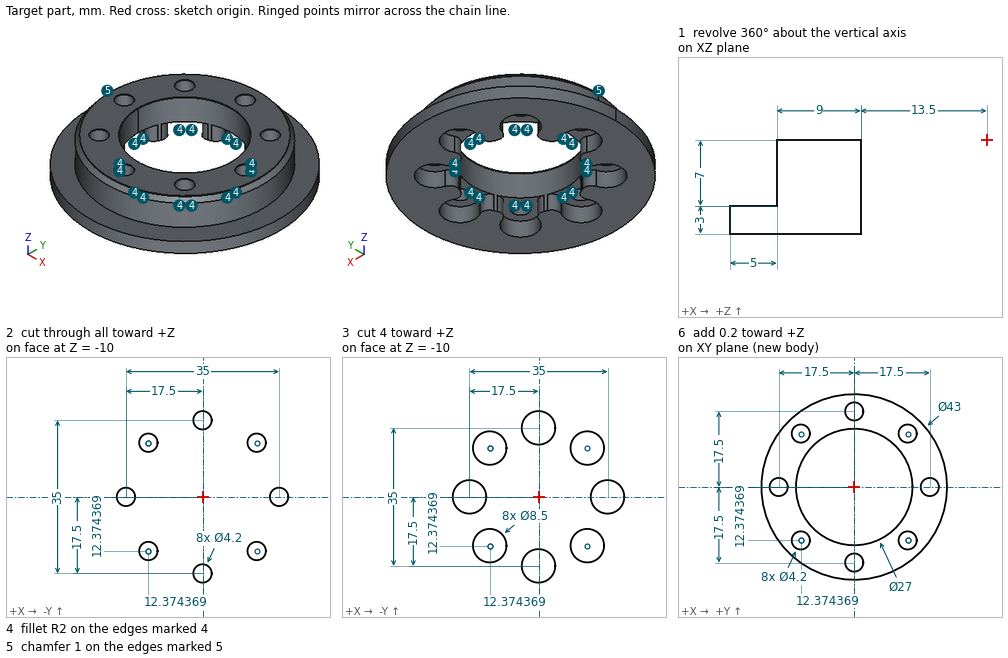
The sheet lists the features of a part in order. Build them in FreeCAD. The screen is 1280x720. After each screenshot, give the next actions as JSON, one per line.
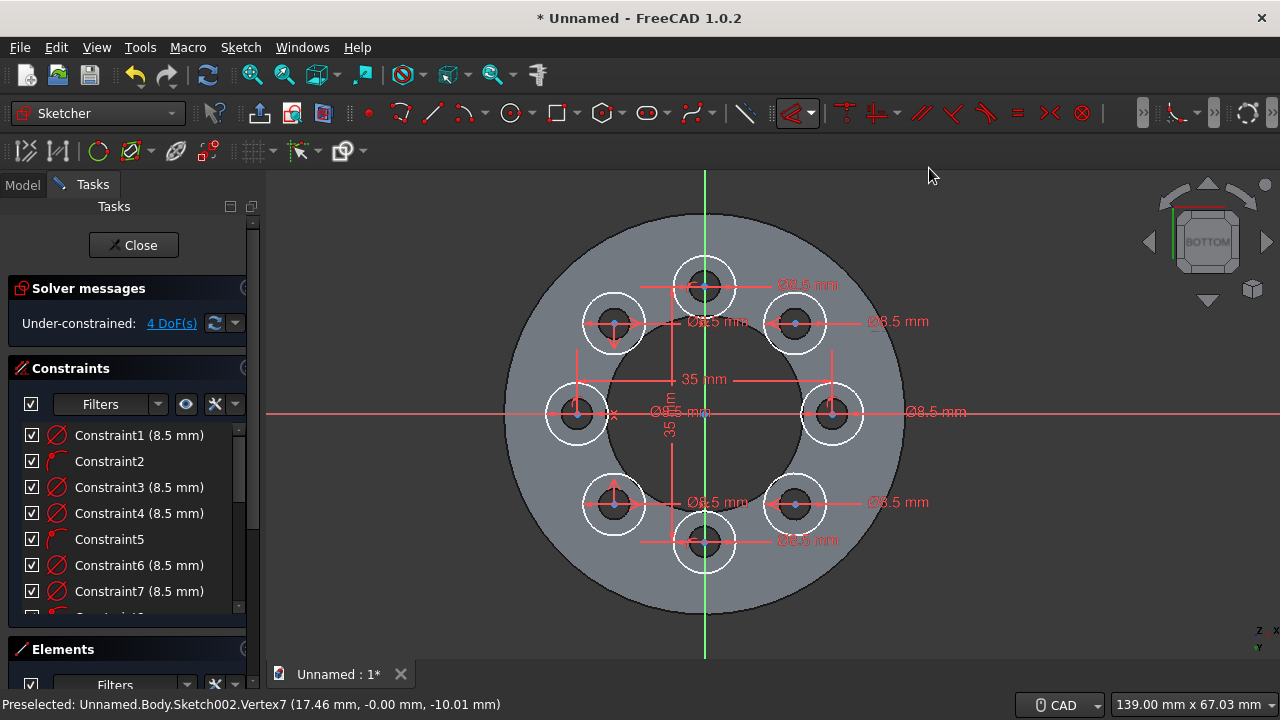
{"action": "left_click", "coordinate": [705, 542]}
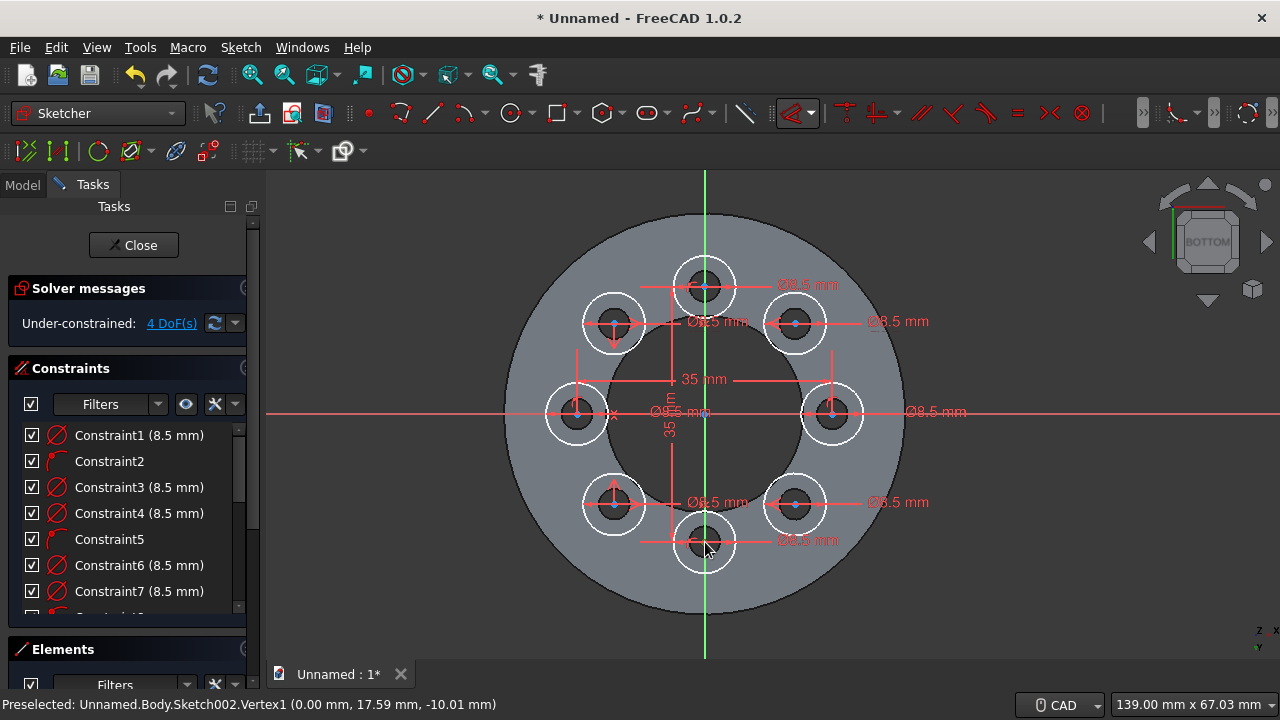
{"action": "key", "text": "i"}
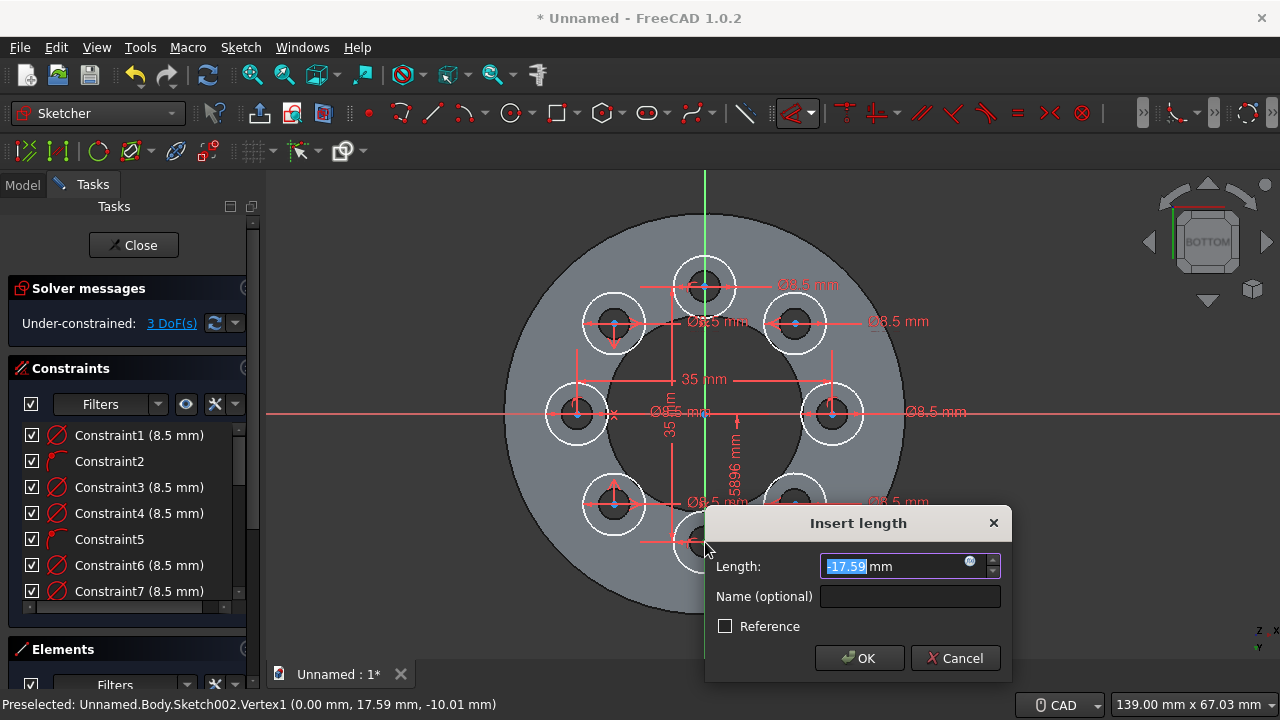
{"action": "type", "text": "-17.5"}
{"action": "key", "text": "Return"}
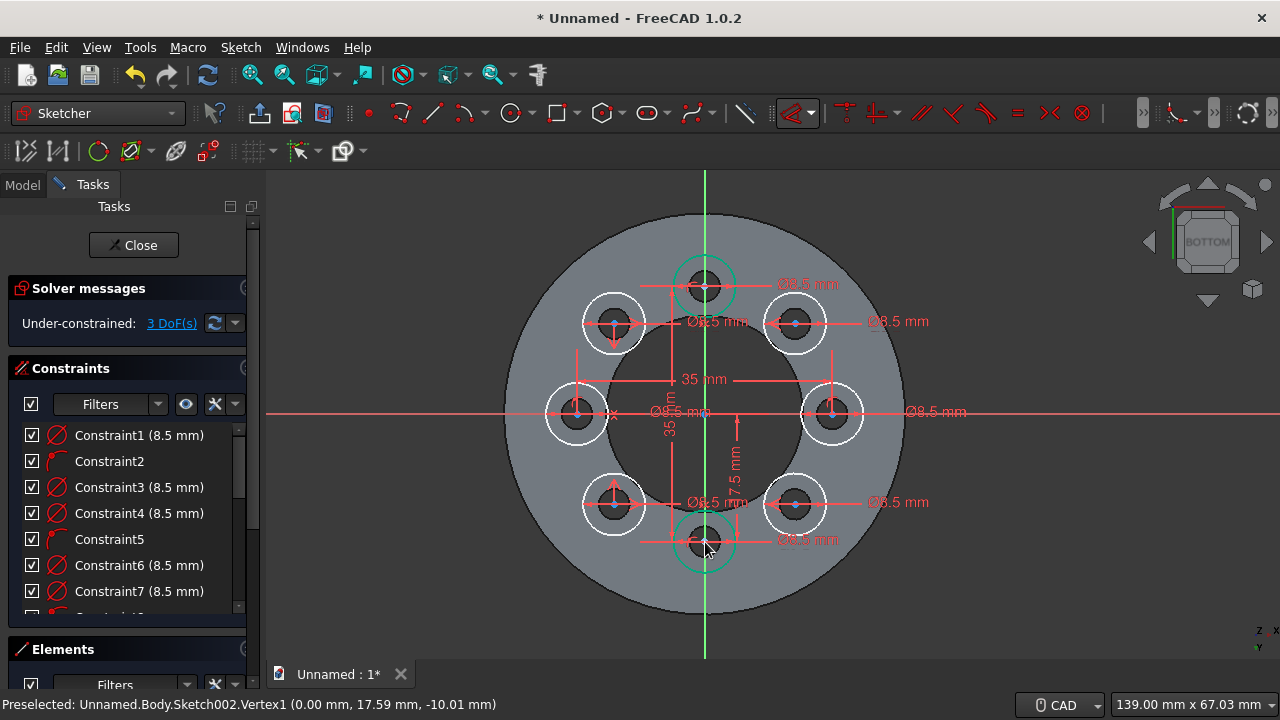
{"action": "left_click", "coordinate": [577, 414]}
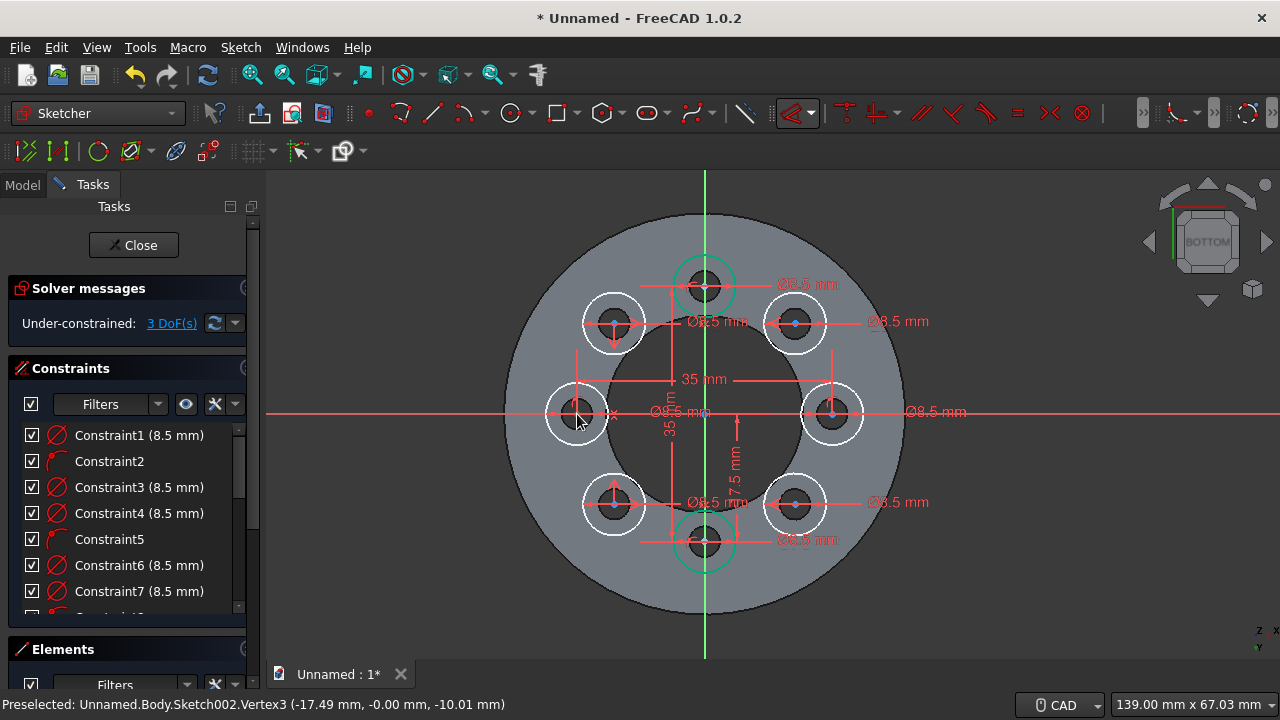
{"action": "key", "text": "l"}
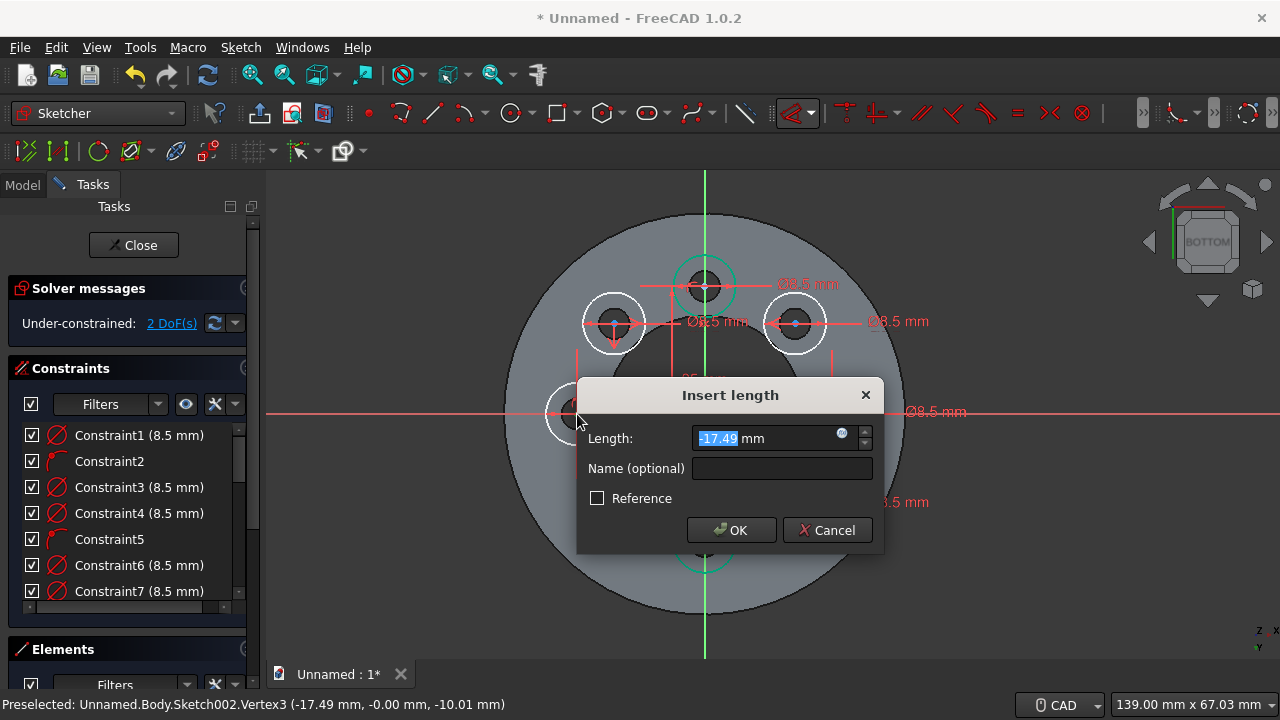
{"action": "type", "text": "-17.5"}
{"action": "key", "text": "Return"}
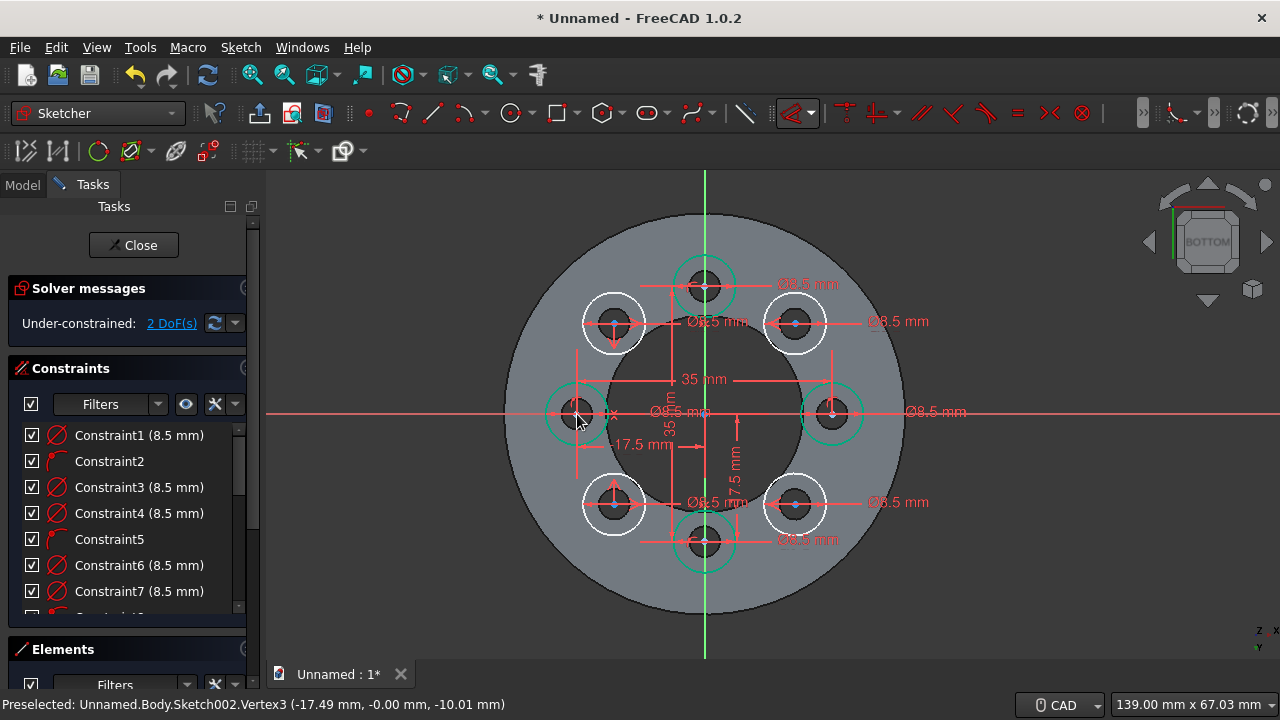
{"action": "left_click", "coordinate": [614, 504]}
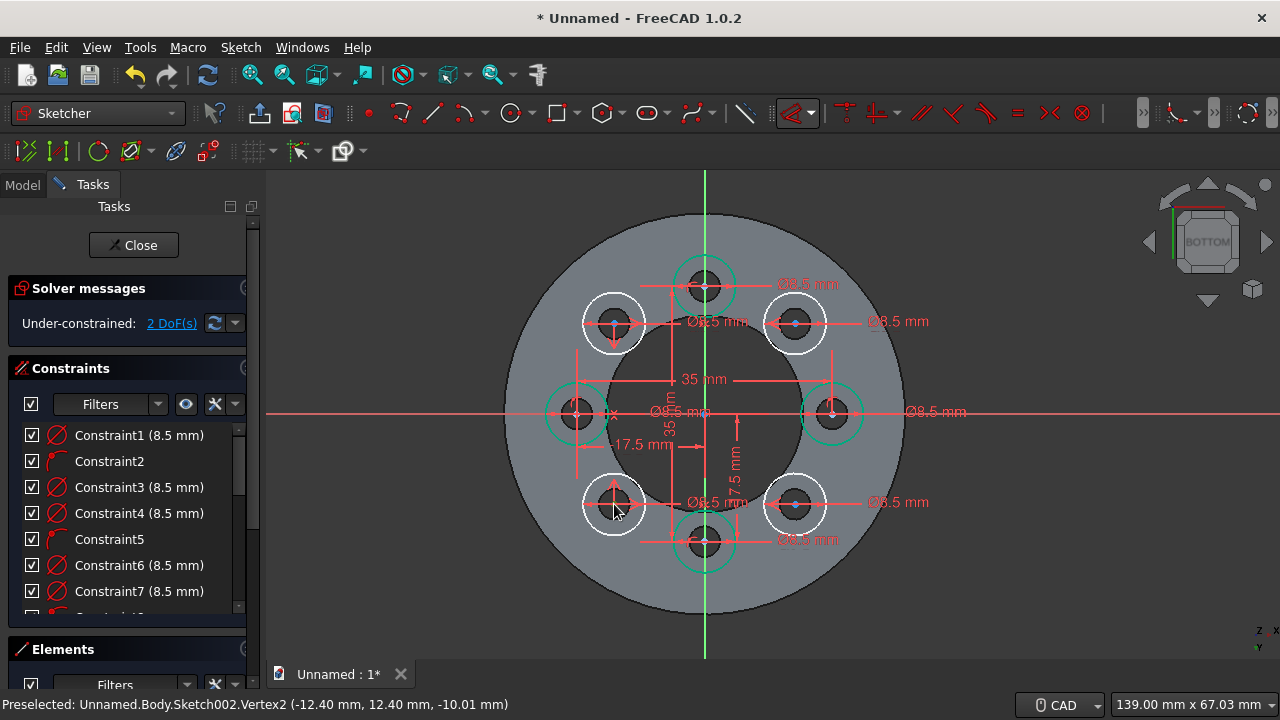
{"action": "left_click", "coordinate": [814, 114]}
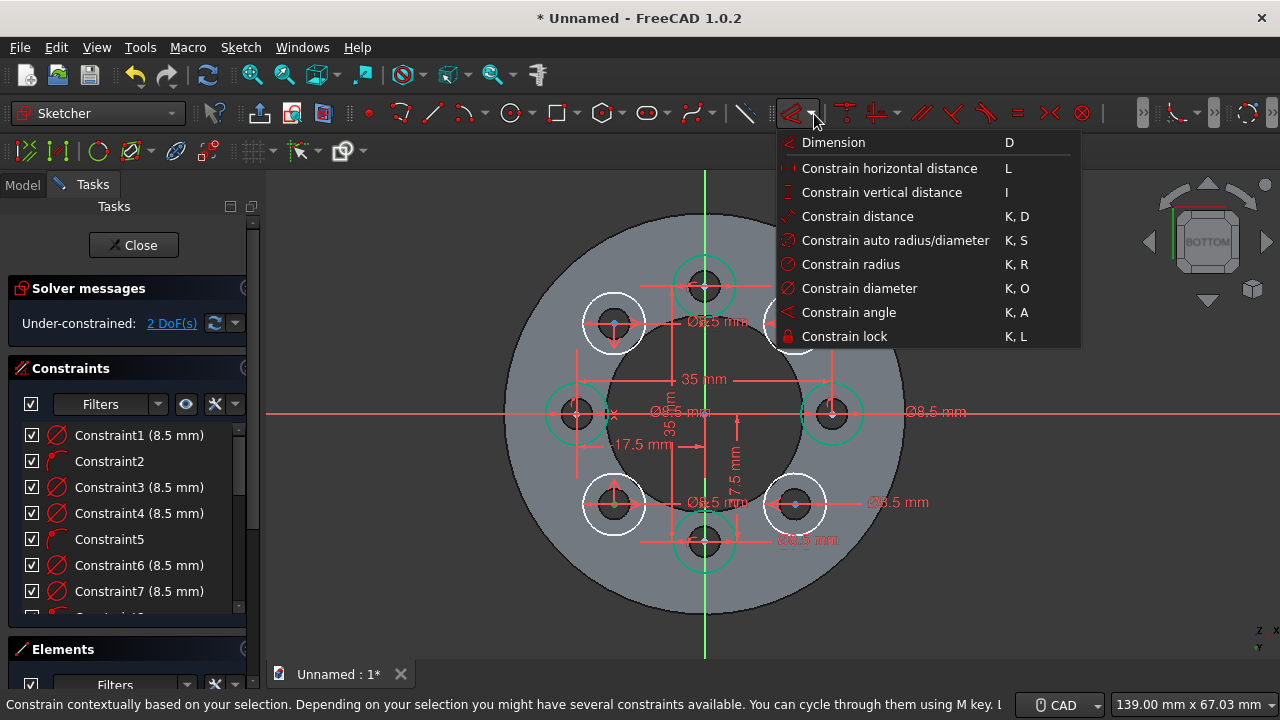
{"action": "left_click", "coordinate": [929, 168]}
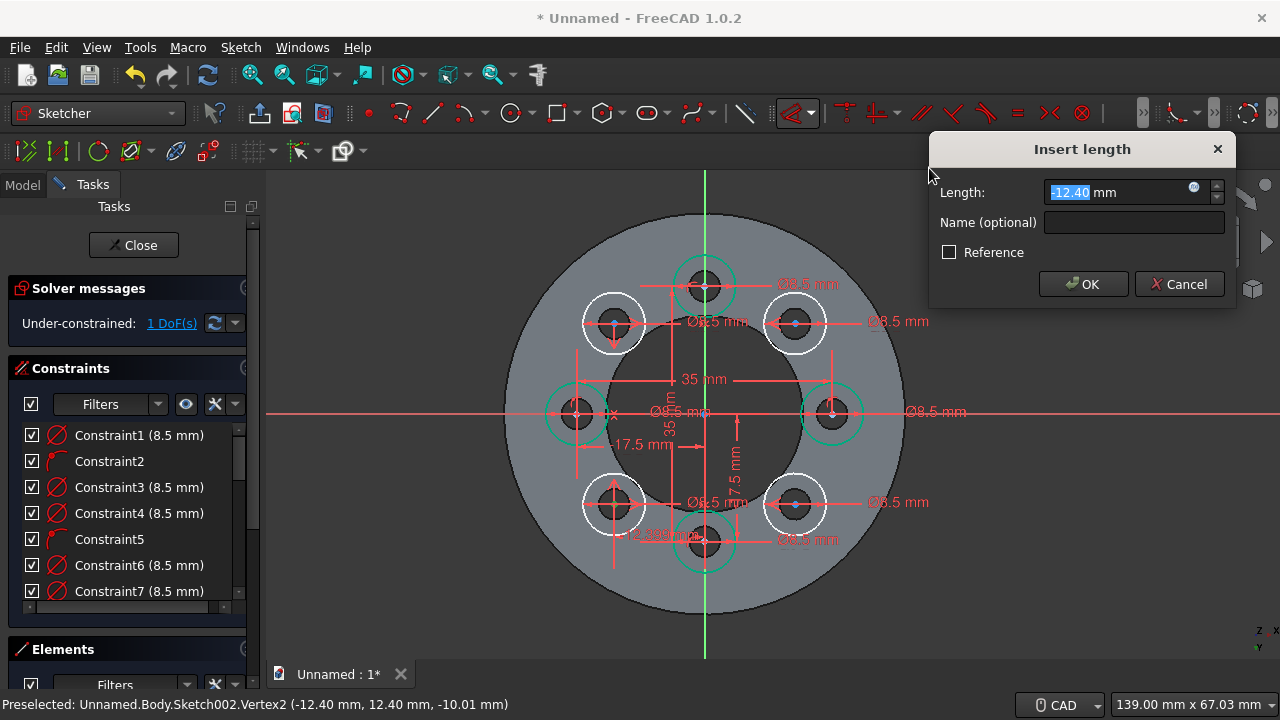
{"action": "type", "text": "-12.374369"}
{"action": "key", "text": "Return"}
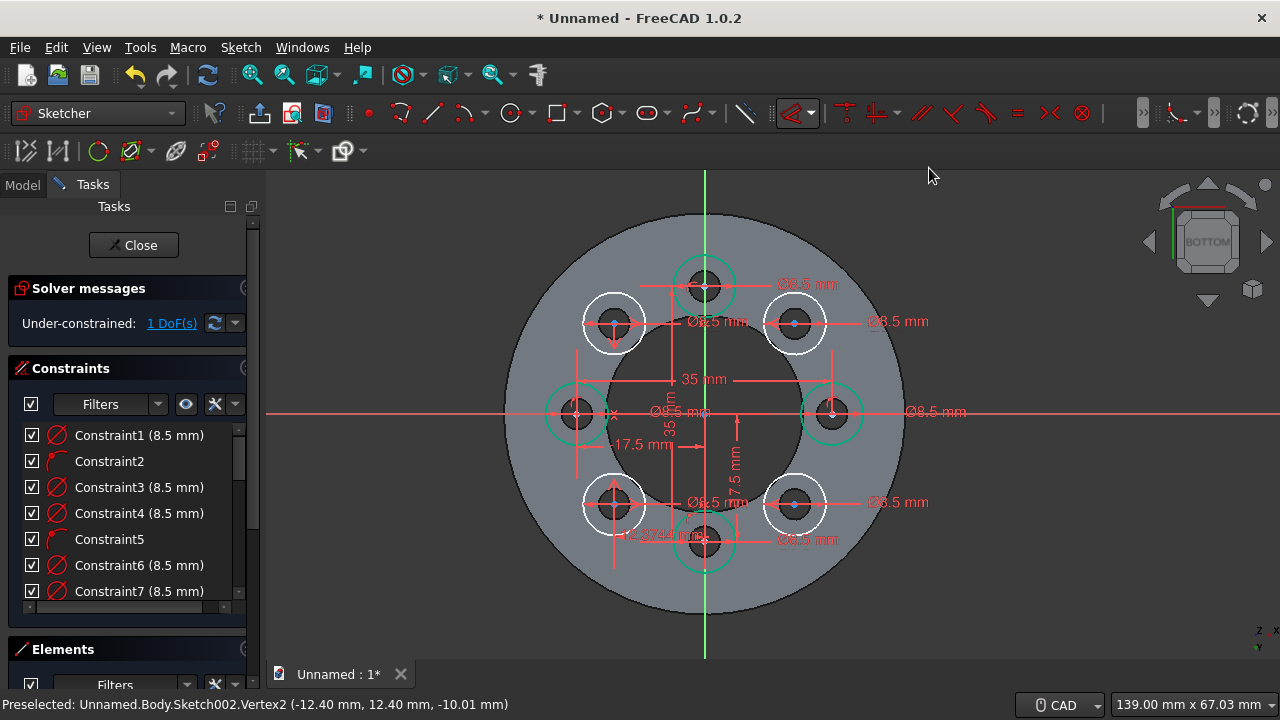
{"action": "left_click", "coordinate": [614, 504]}